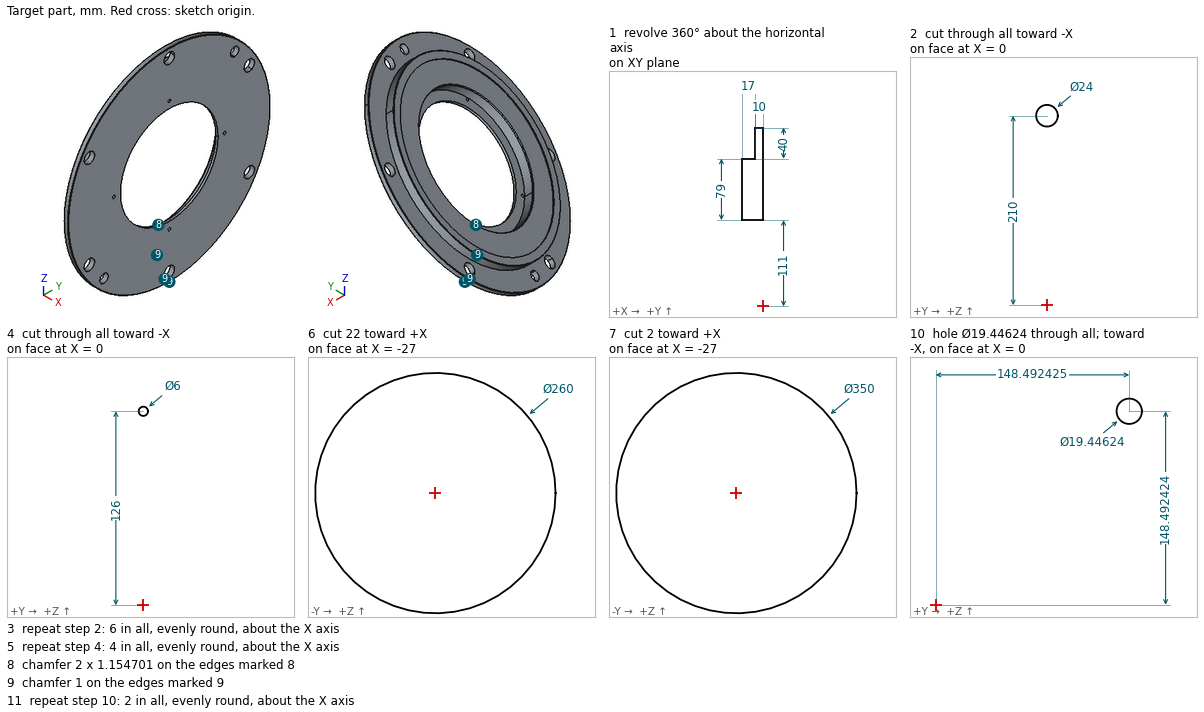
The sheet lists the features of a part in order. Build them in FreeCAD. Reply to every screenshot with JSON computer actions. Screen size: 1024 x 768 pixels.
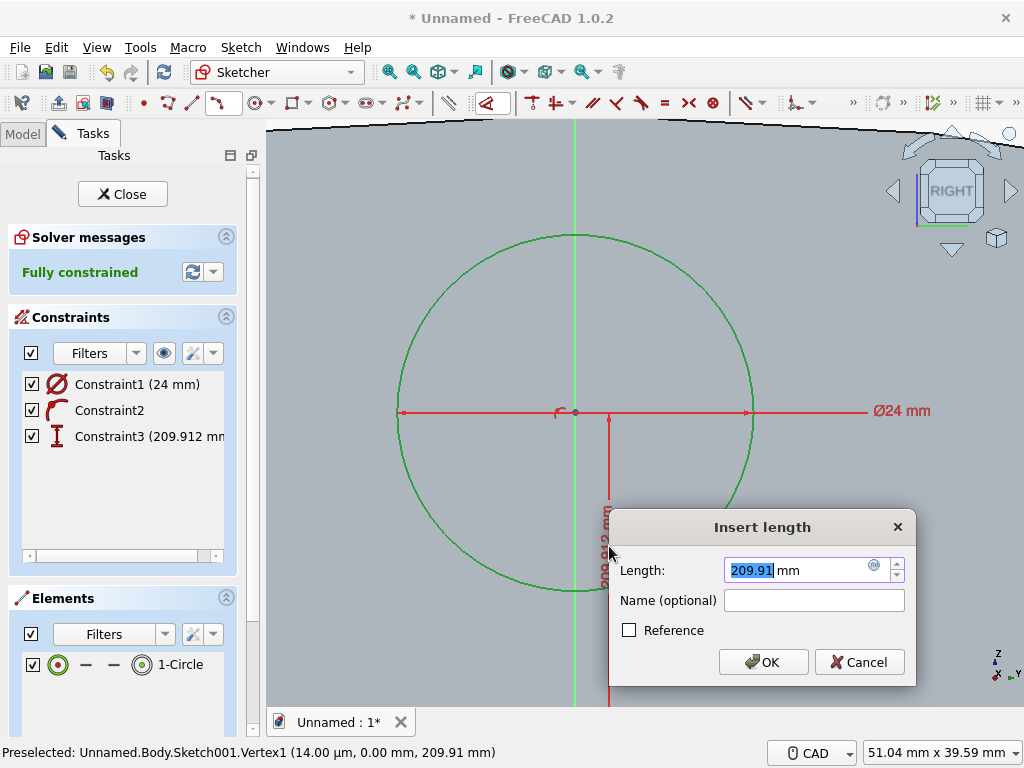
{"action": "type", "text": "210"}
{"action": "key", "text": "Return"}
{"action": "key", "text": "Escape"}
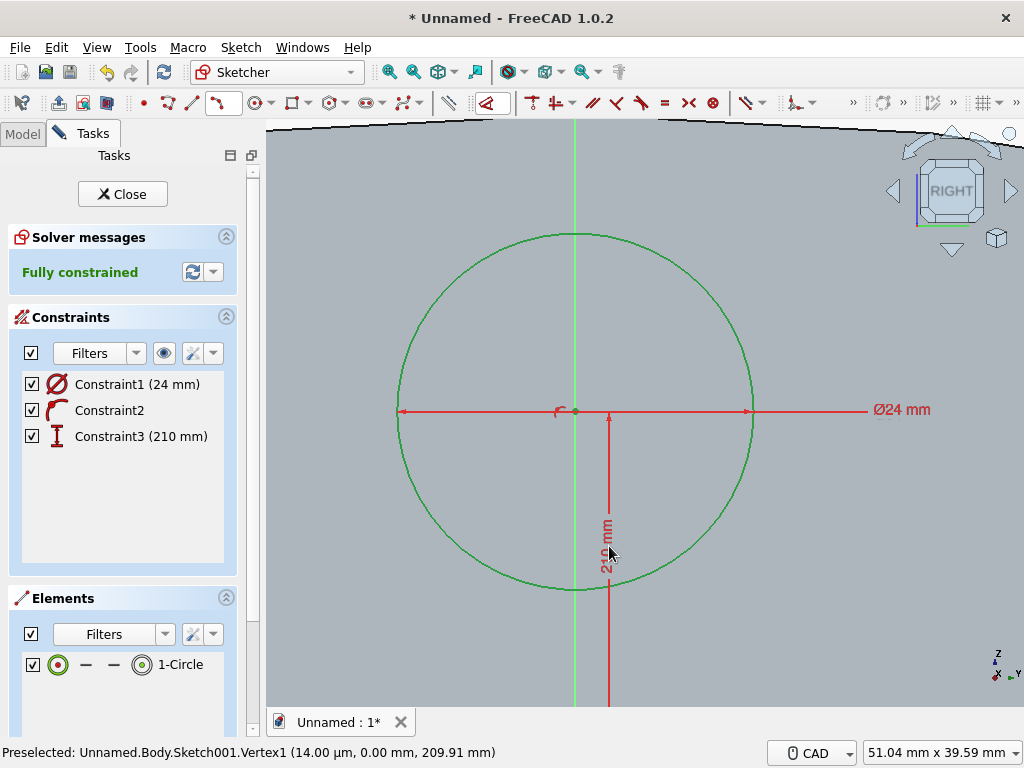
{"action": "left_click", "coordinate": [123, 194]}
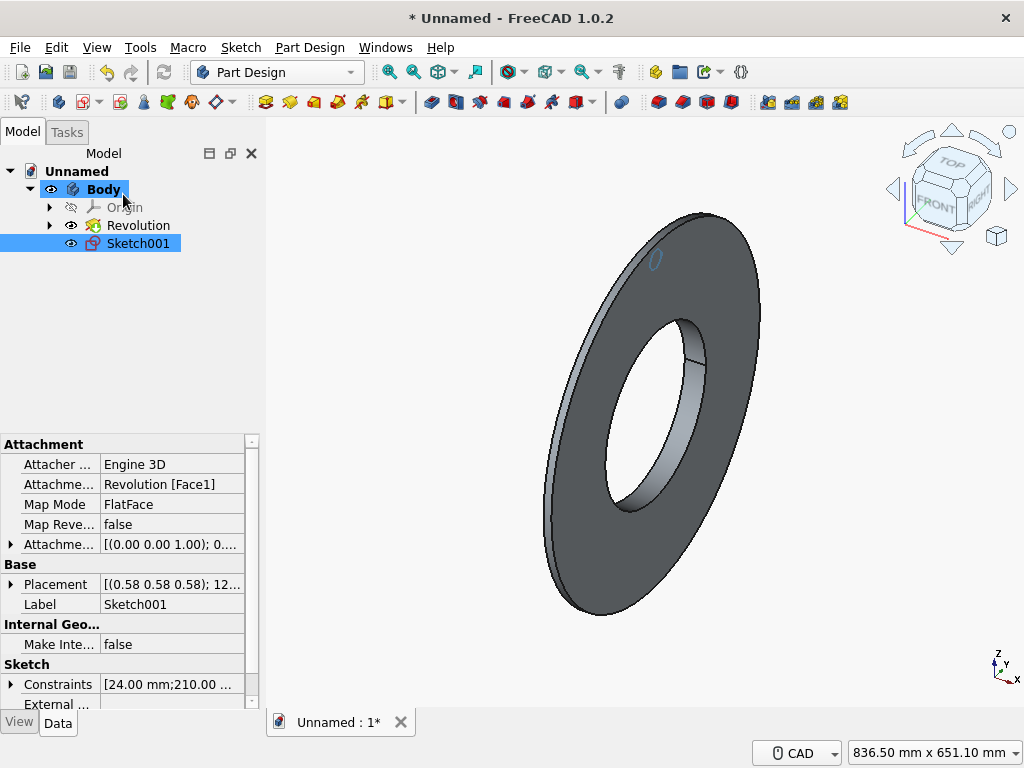
{"action": "left_click", "coordinate": [432, 102]}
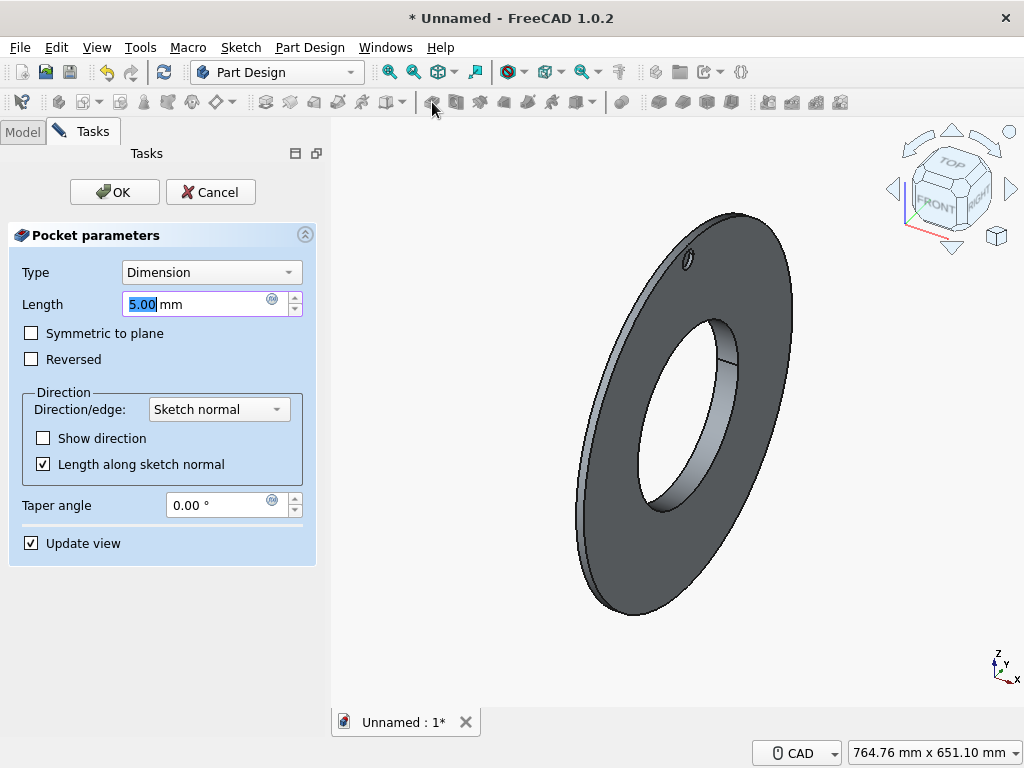
{"action": "left_click", "coordinate": [212, 272]}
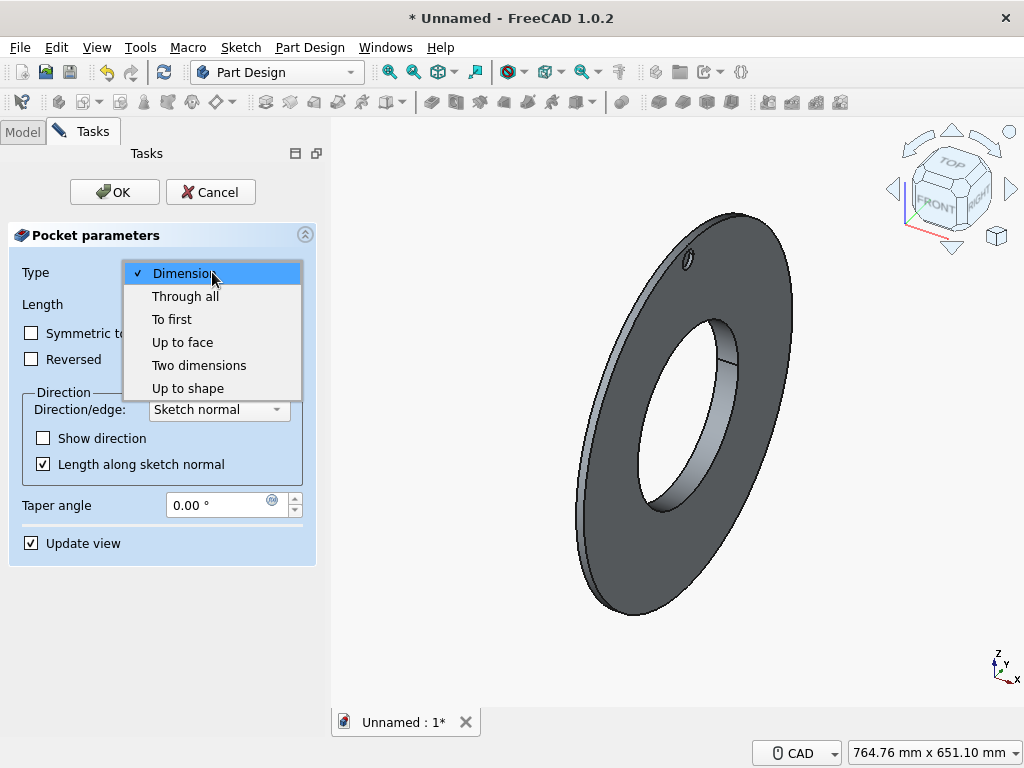
{"action": "left_click", "coordinate": [212, 296]}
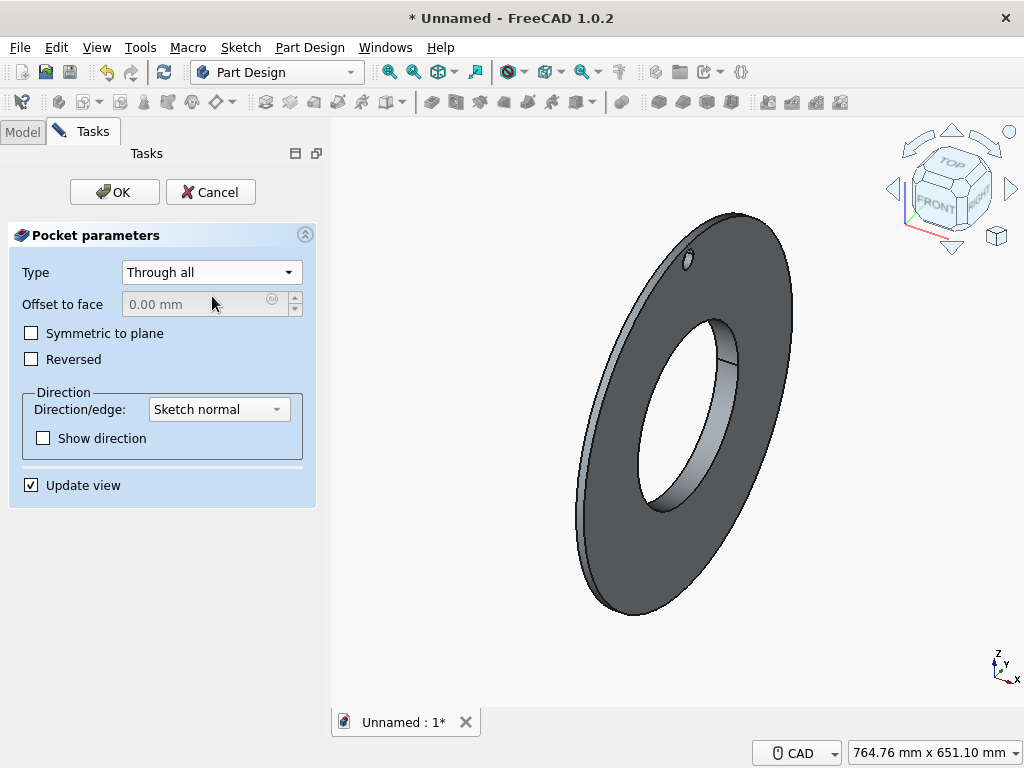
{"action": "left_click", "coordinate": [115, 192]}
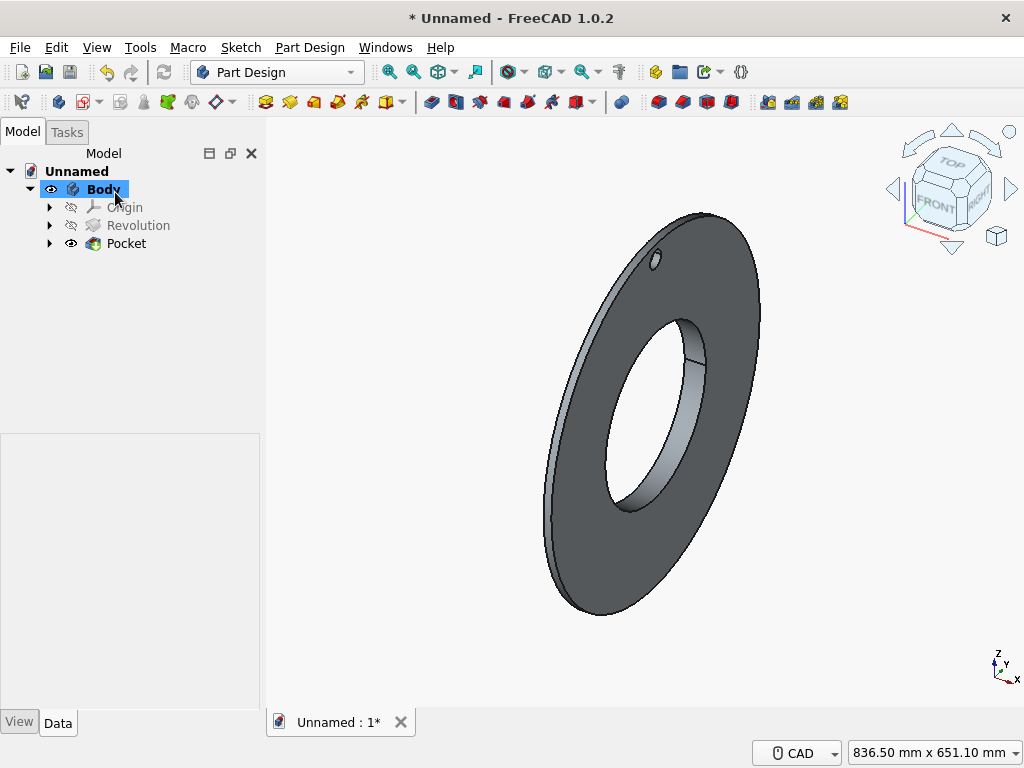
{"action": "left_click", "coordinate": [116, 243]}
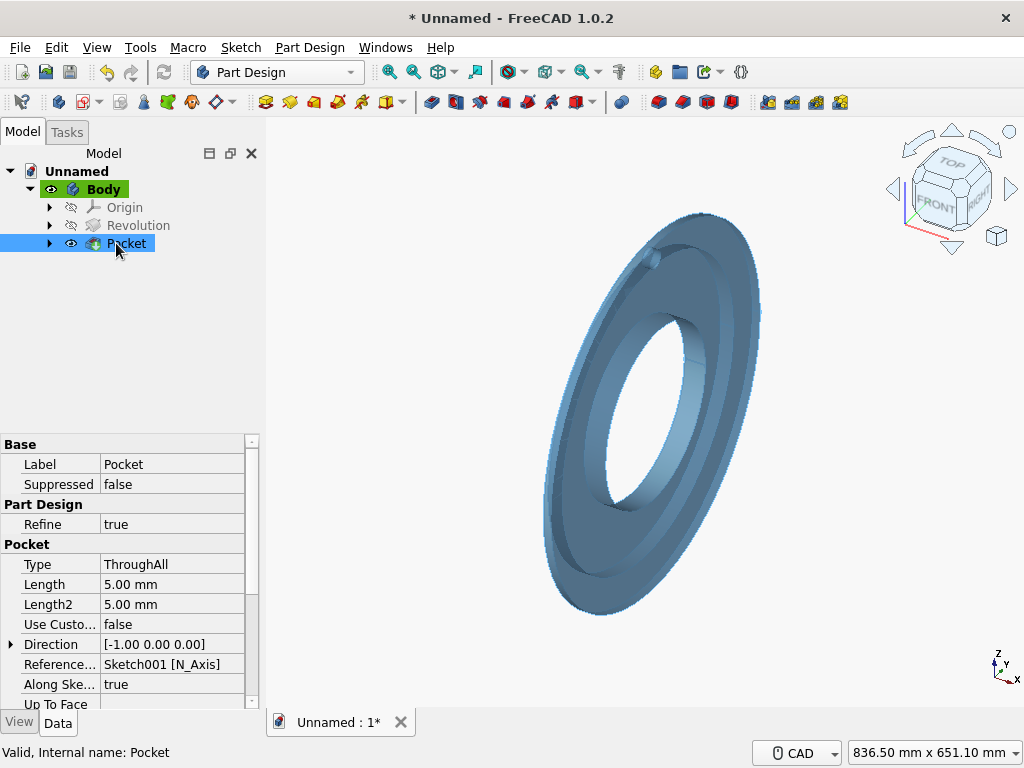
{"action": "left_click", "coordinate": [816, 102]}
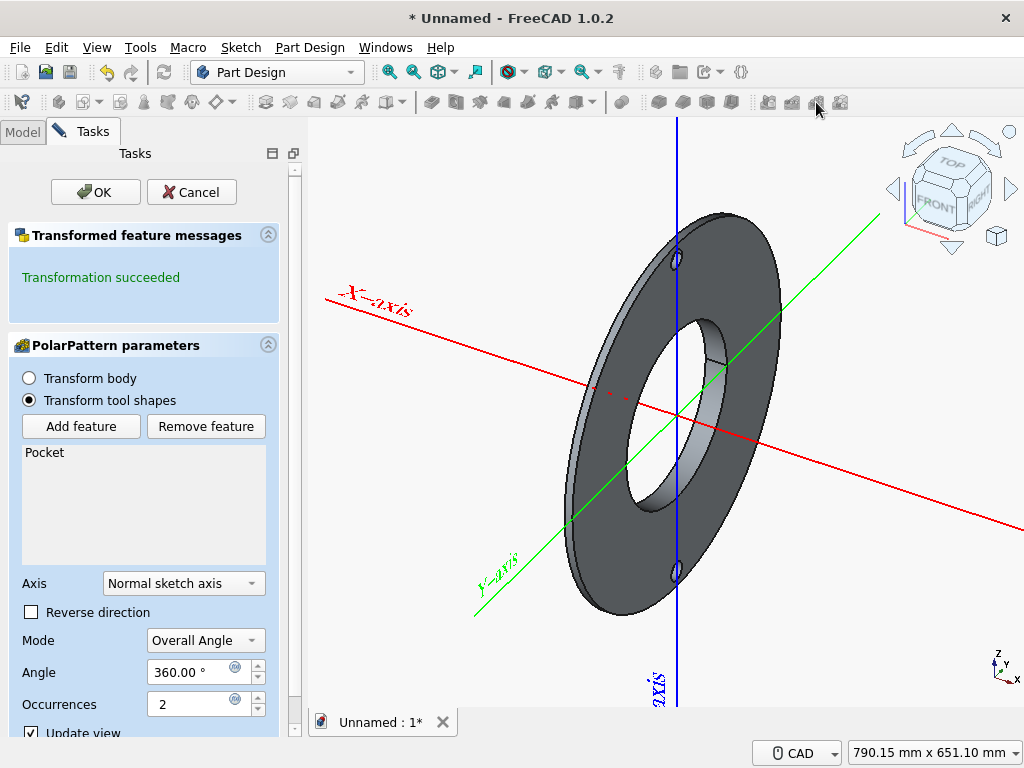
{"action": "left_click", "coordinate": [184, 584]}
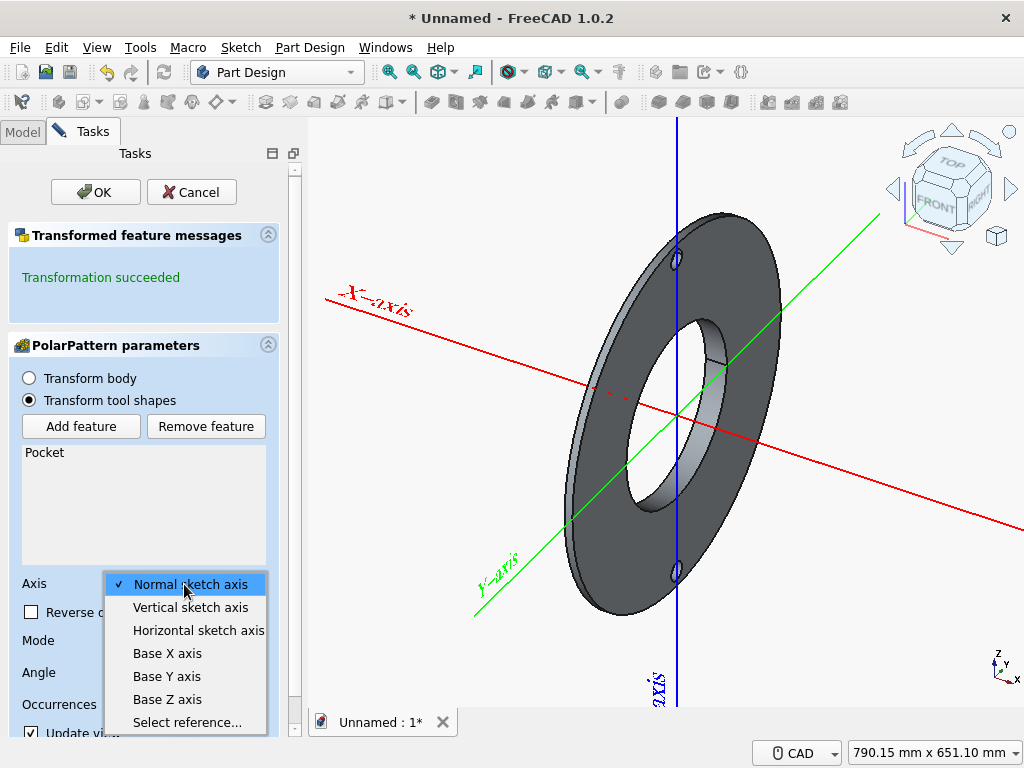
{"action": "left_click", "coordinate": [184, 654]}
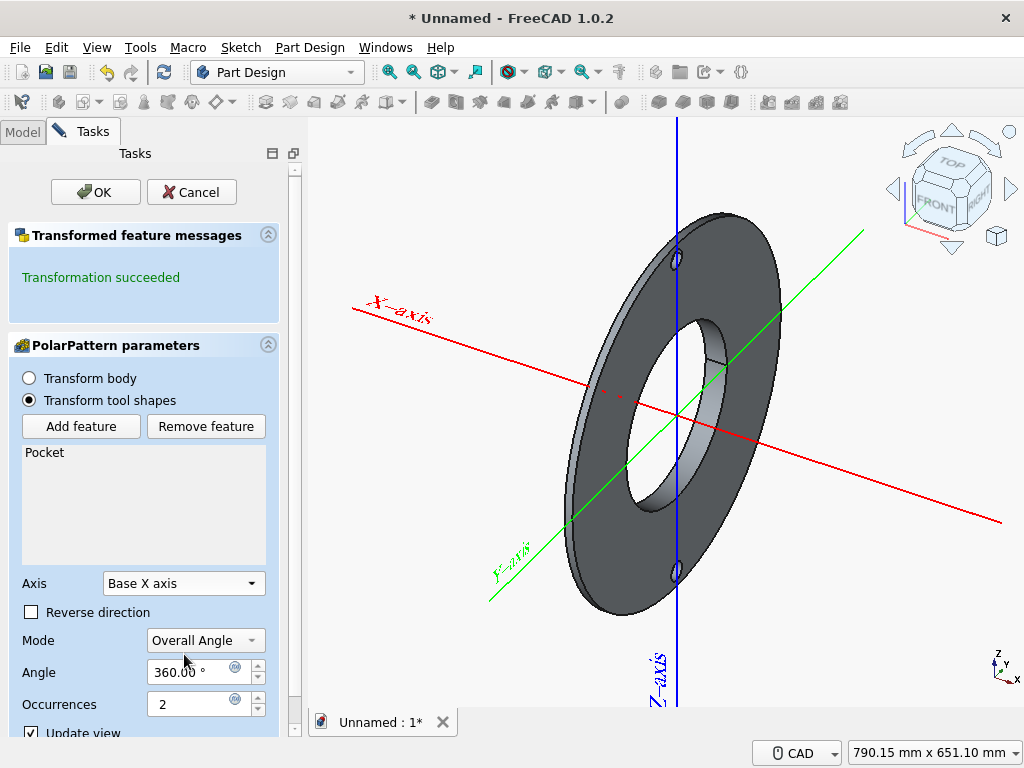
{"action": "triple_click", "coordinate": [198, 704]}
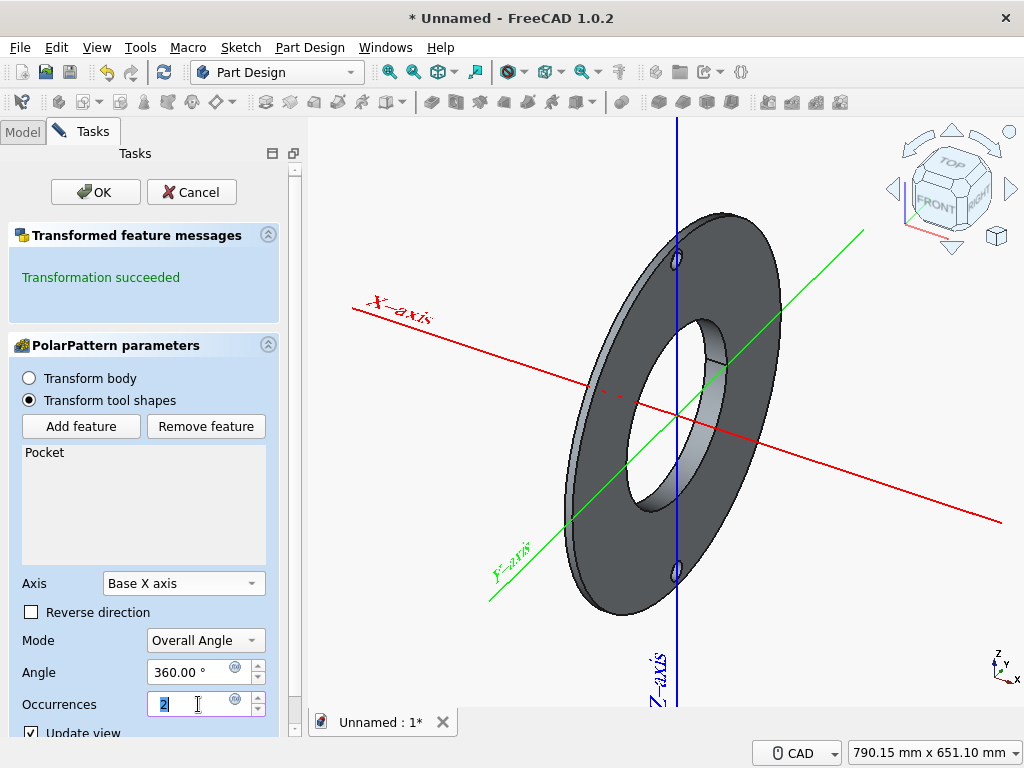
{"action": "type", "text": "6"}
{"action": "key", "text": "Tab"}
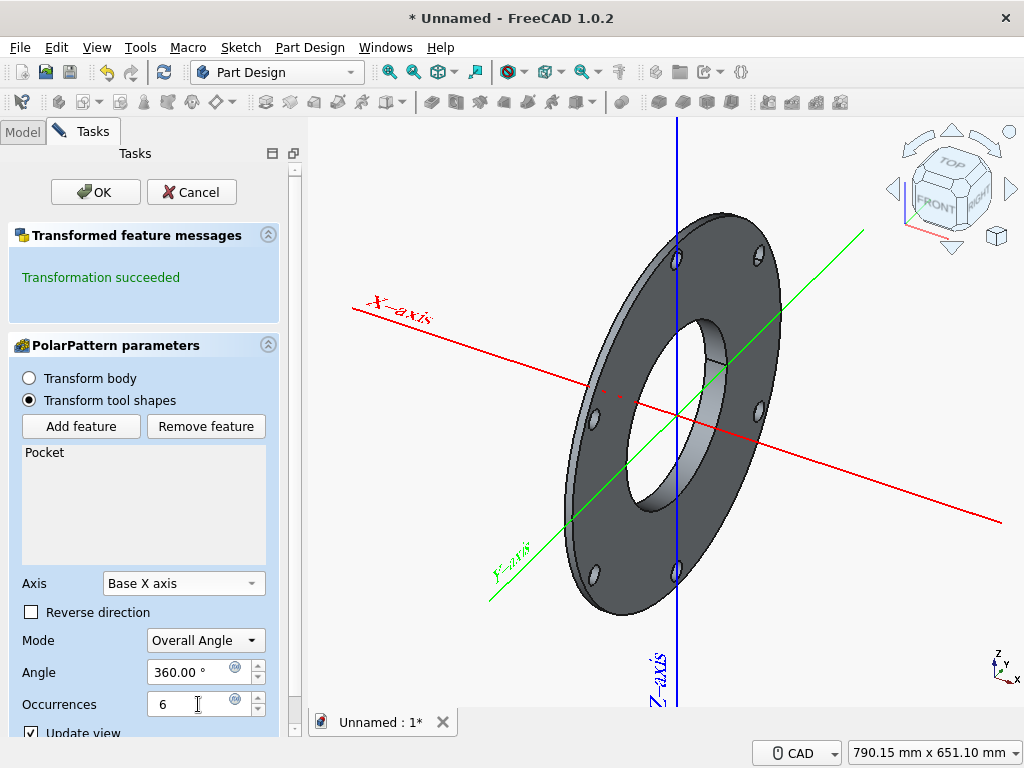
{"action": "left_click", "coordinate": [96, 192]}